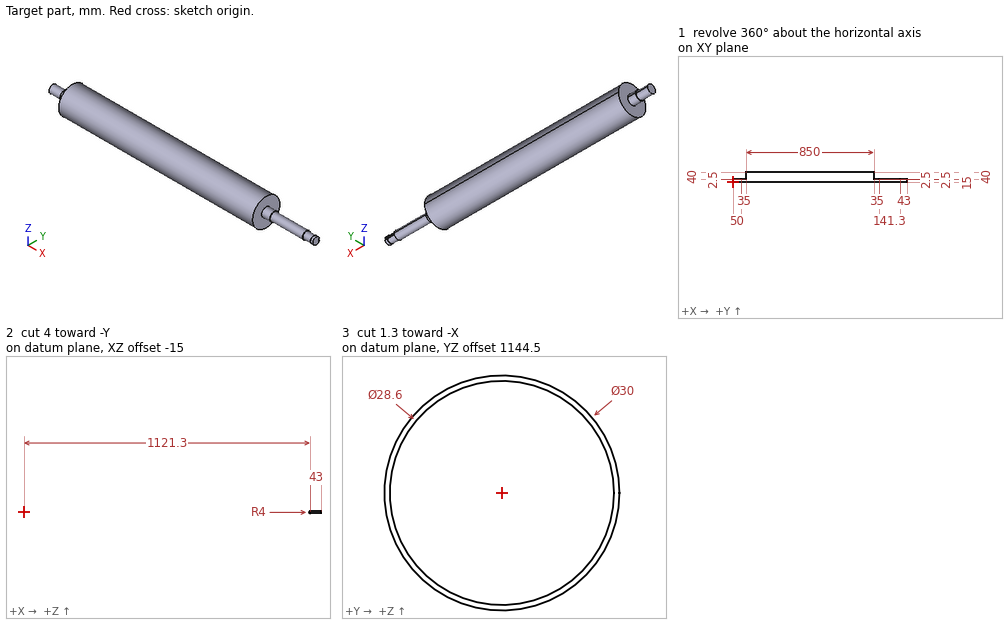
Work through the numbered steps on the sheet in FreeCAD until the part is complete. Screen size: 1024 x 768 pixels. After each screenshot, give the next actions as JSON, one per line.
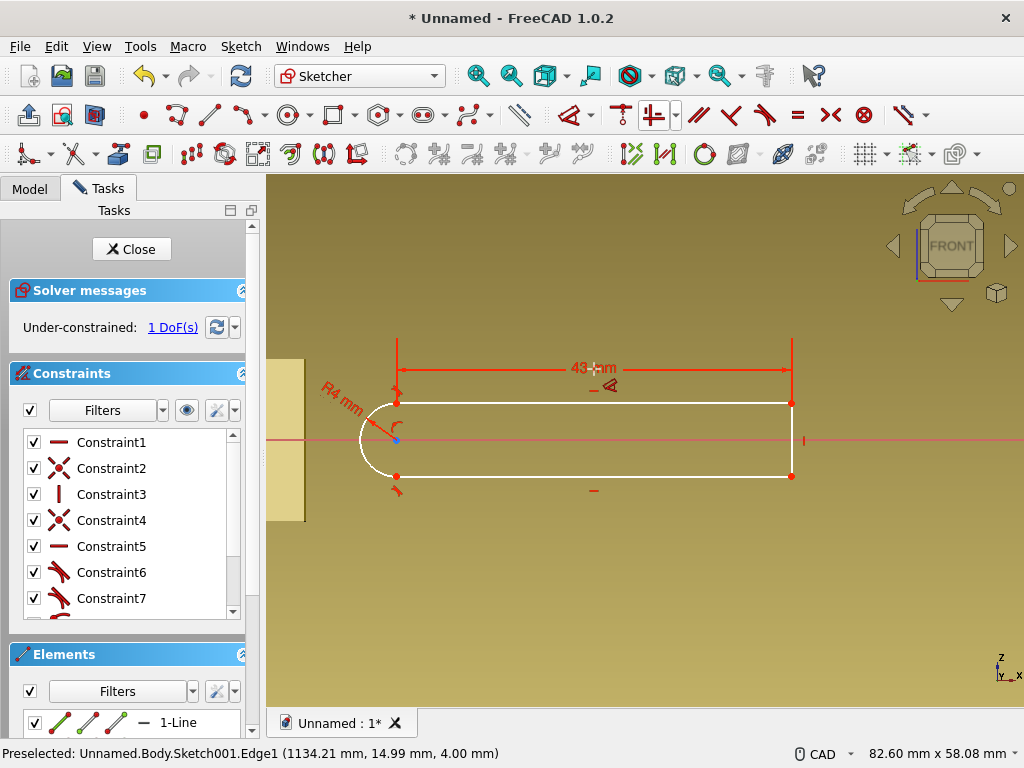
{"action": "left_click", "coordinate": [397, 403]}
{"action": "left_click", "coordinate": [346, 369]}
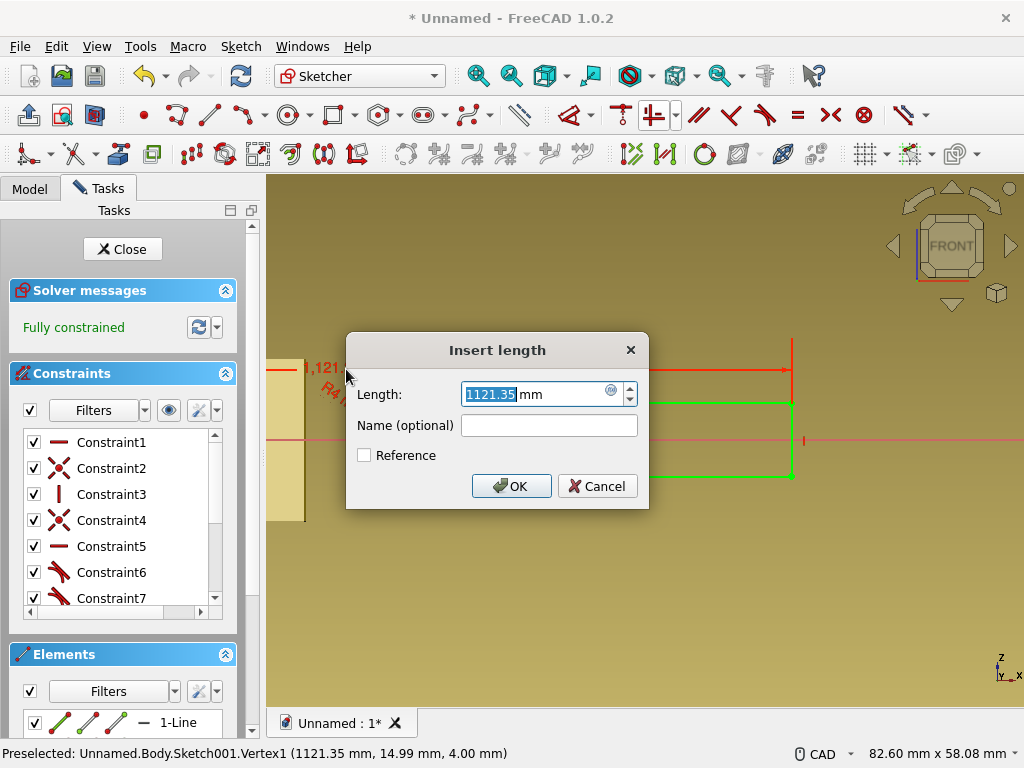
{"action": "type", "text": "1121.3"}
{"action": "key", "text": "Return"}
{"action": "key", "text": "Escape"}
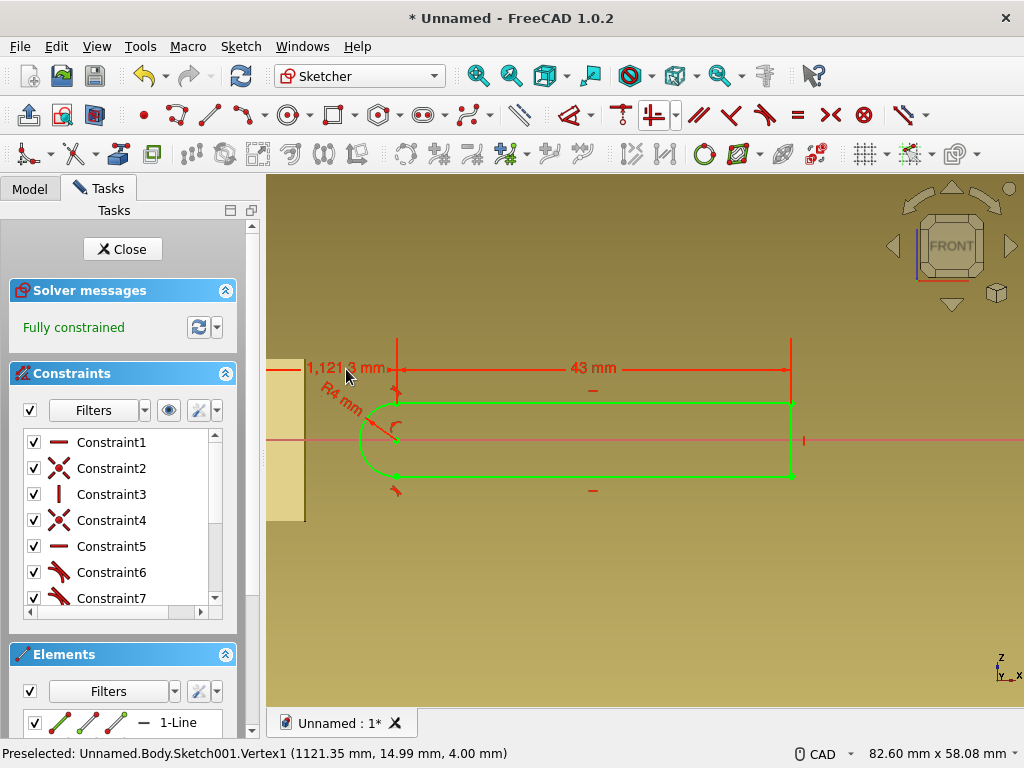
{"action": "left_click", "coordinate": [123, 249]}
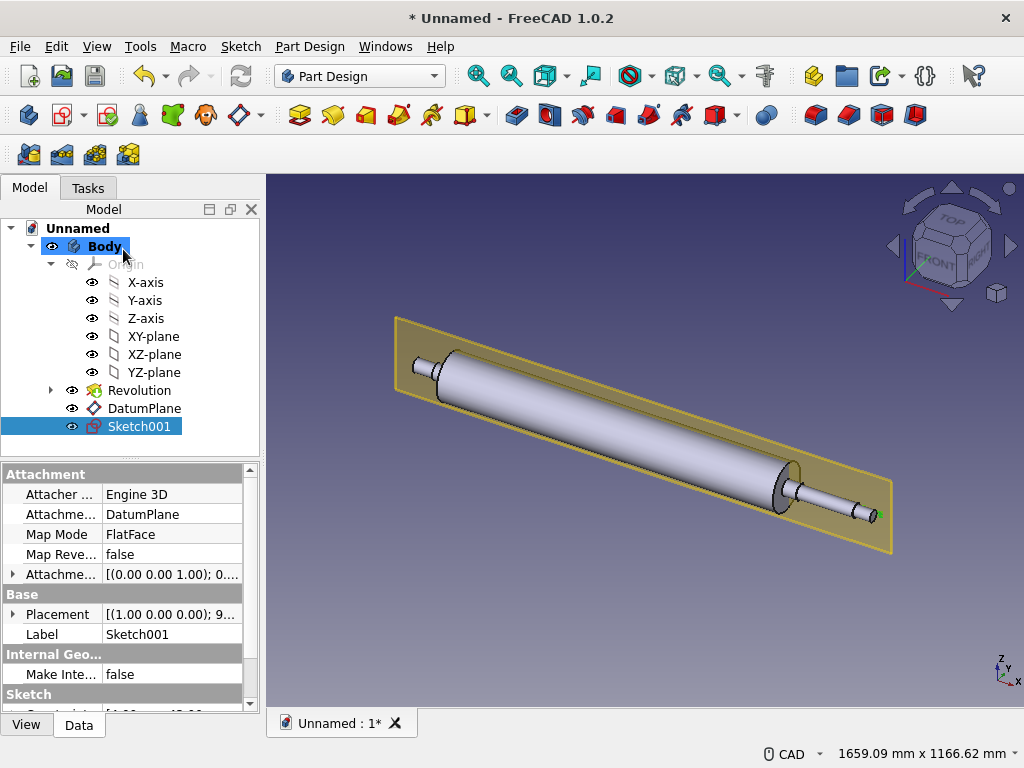
{"action": "left_click", "coordinate": [517, 116]}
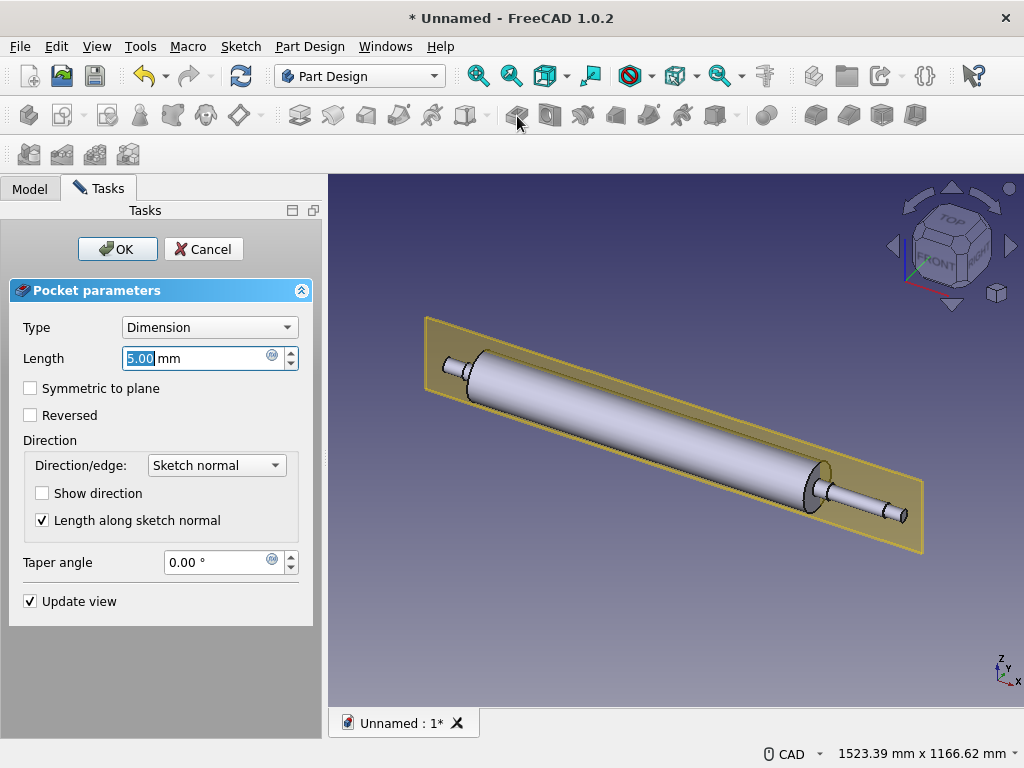
{"action": "type", "text": "4"}
{"action": "key", "text": "Tab"}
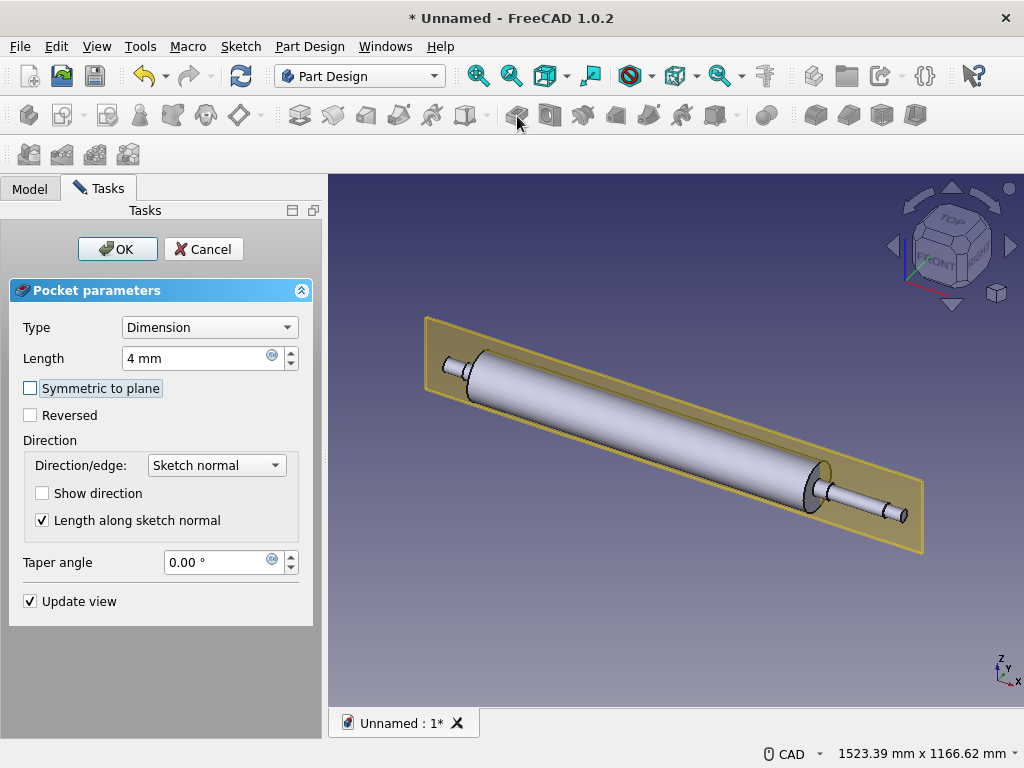
{"action": "left_click", "coordinate": [31, 415]}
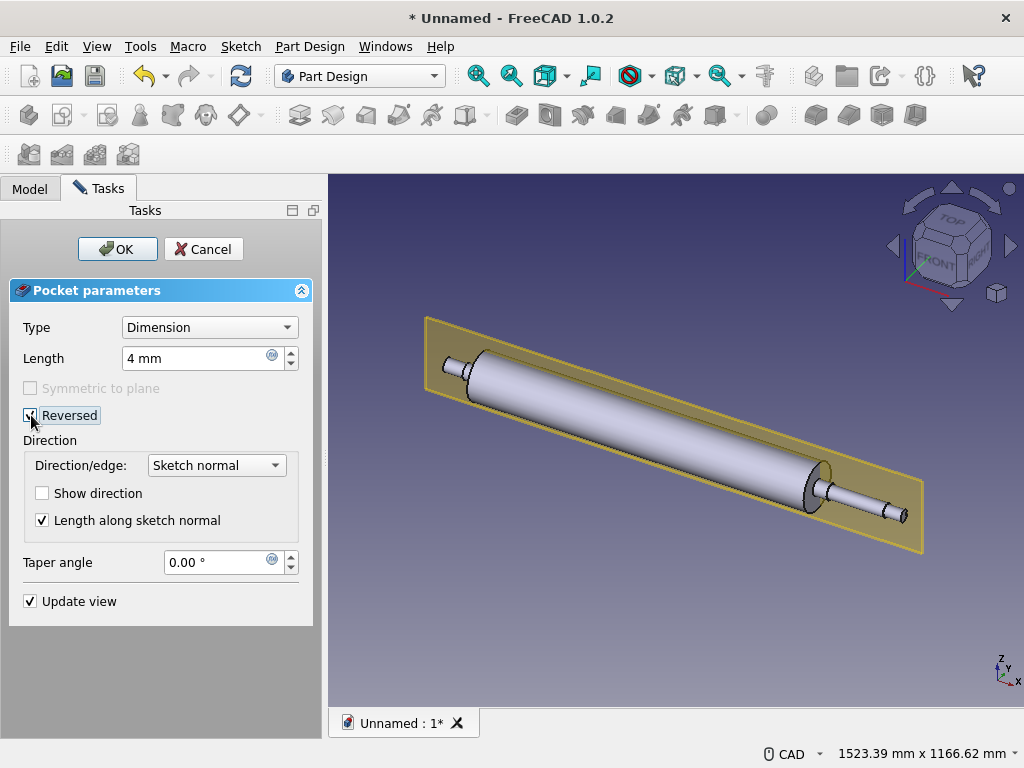
{"action": "left_click", "coordinate": [118, 249]}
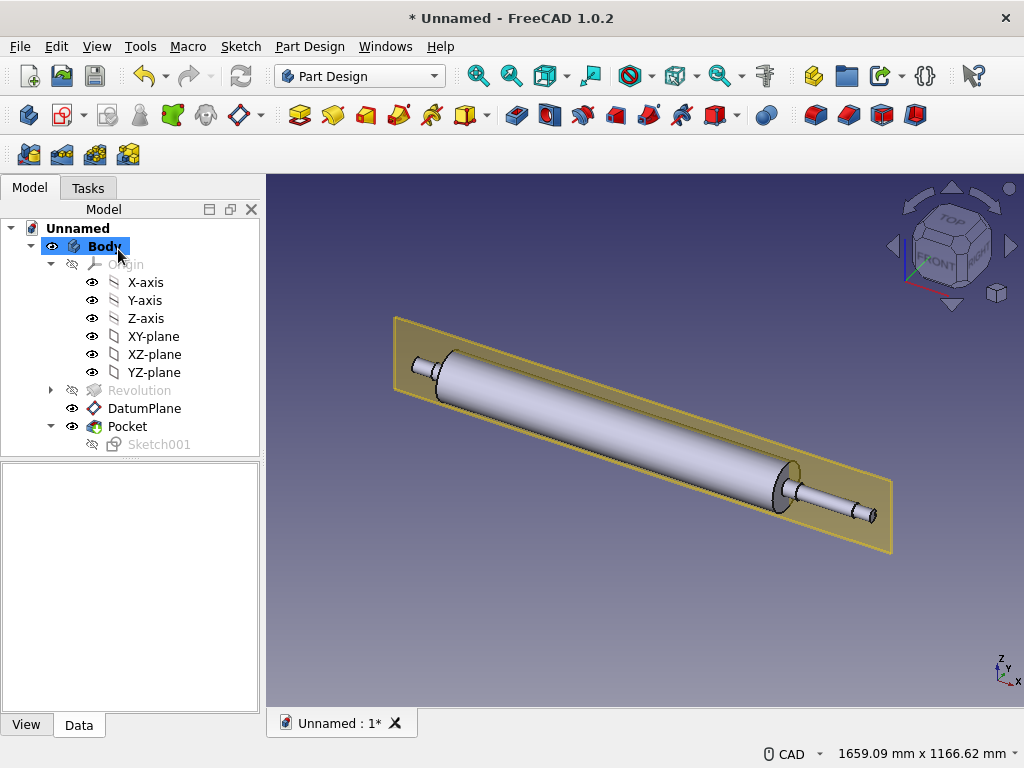
{"action": "left_click", "coordinate": [117, 408]}
{"action": "key", "text": "space"}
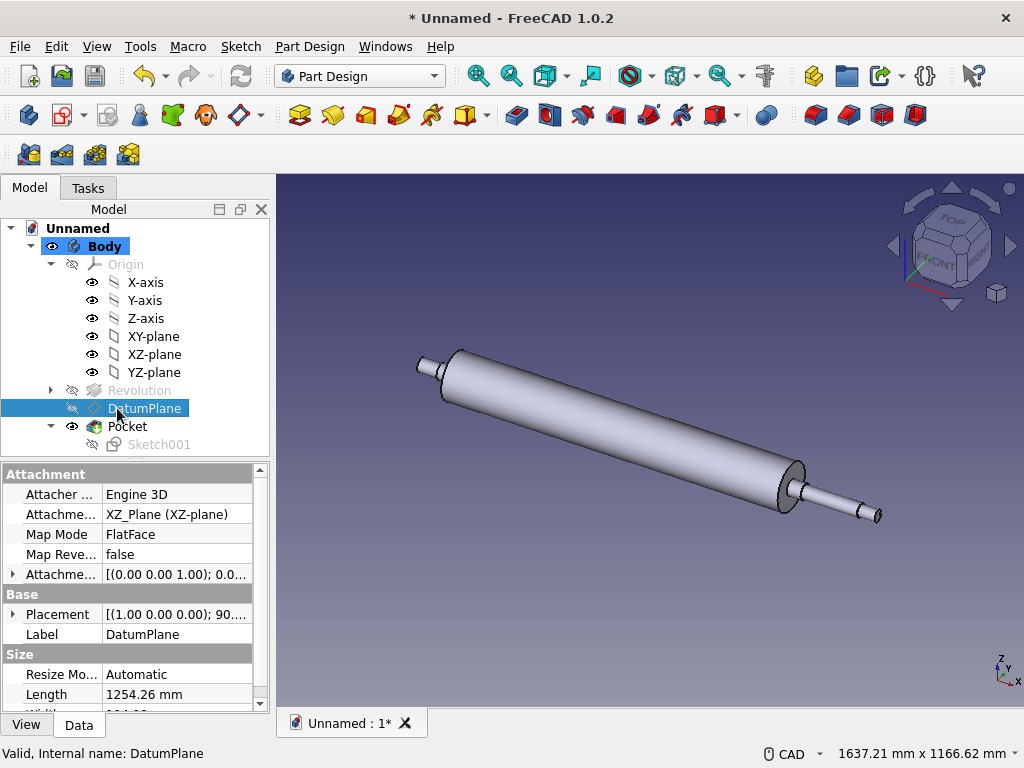
{"action": "left_click", "coordinate": [137, 372]}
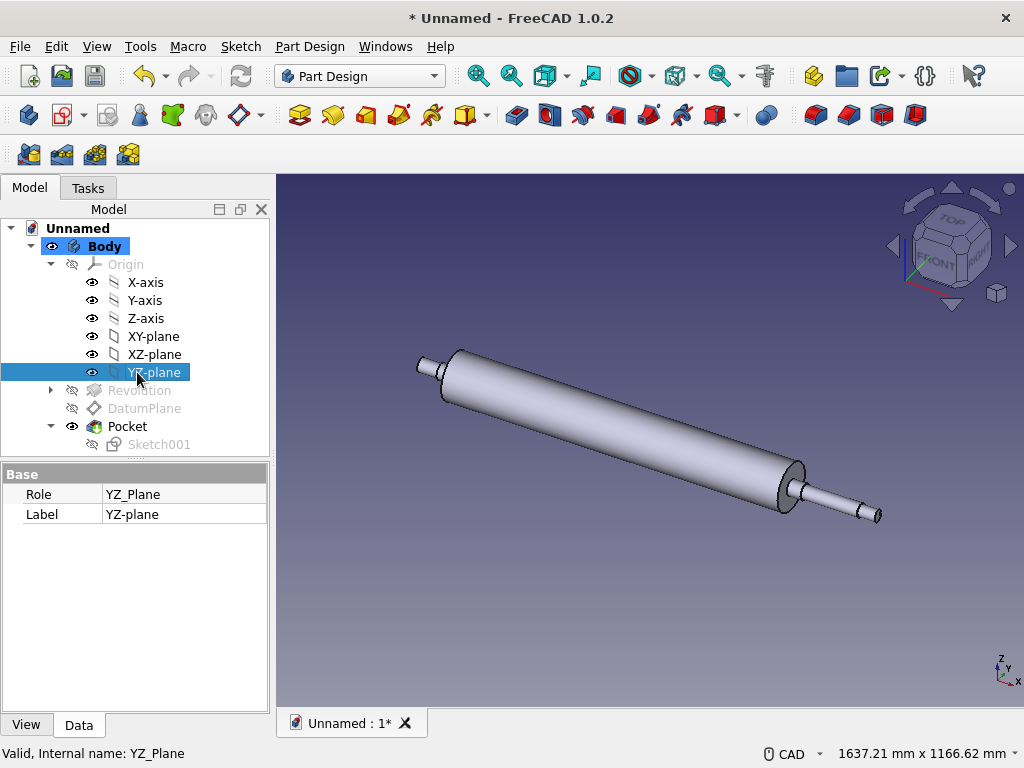
{"action": "left_click", "coordinate": [238, 116]}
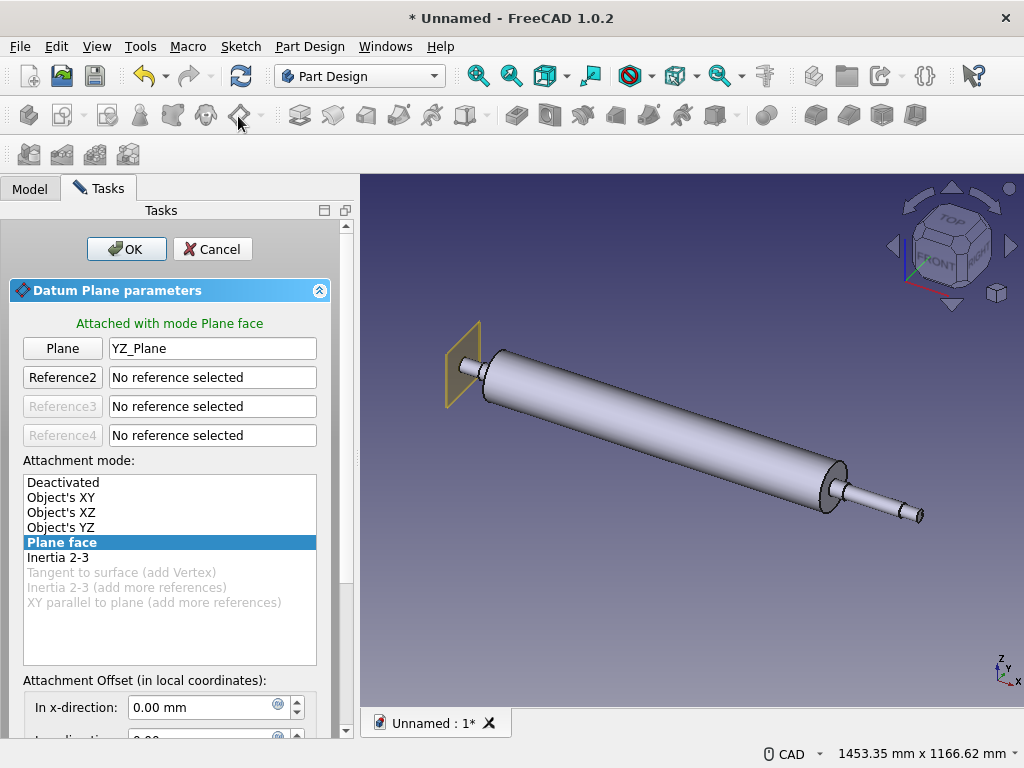
{"action": "scroll", "coordinate": [346, 479], "scroll_direction": "down", "scroll_amount": 2}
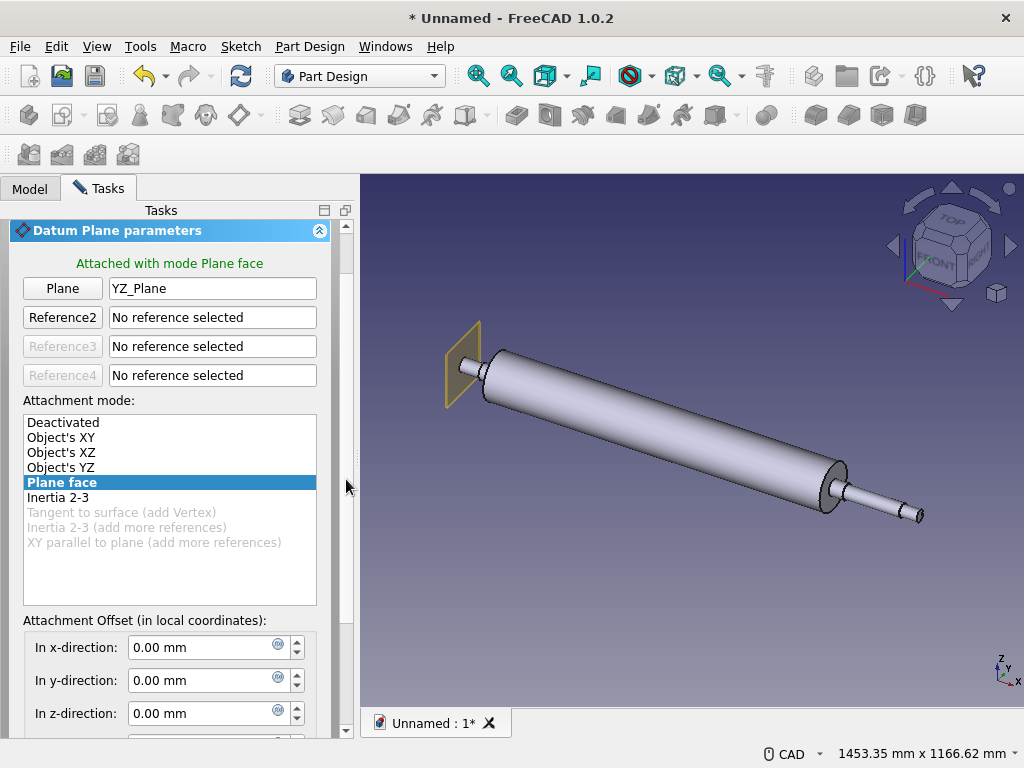
{"action": "triple_click", "coordinate": [210, 654]}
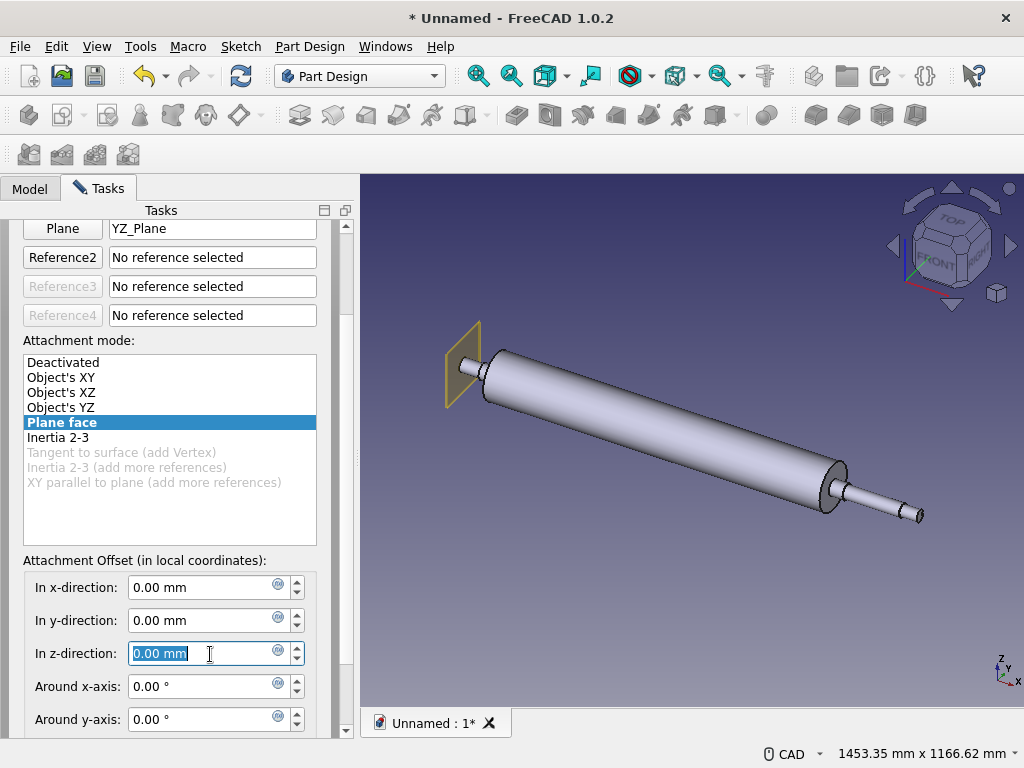
{"action": "type", "text": "1144.5"}
{"action": "key", "text": "Tab"}